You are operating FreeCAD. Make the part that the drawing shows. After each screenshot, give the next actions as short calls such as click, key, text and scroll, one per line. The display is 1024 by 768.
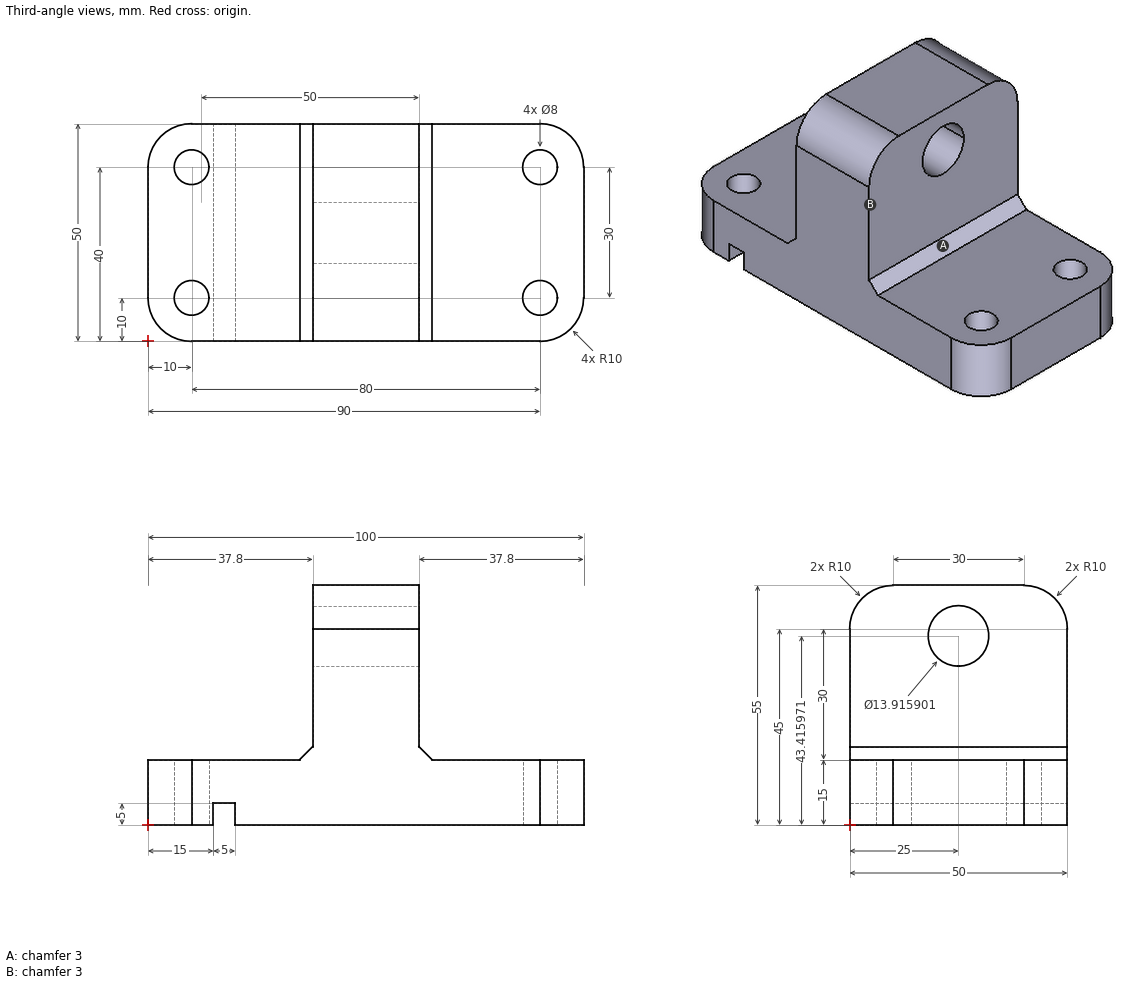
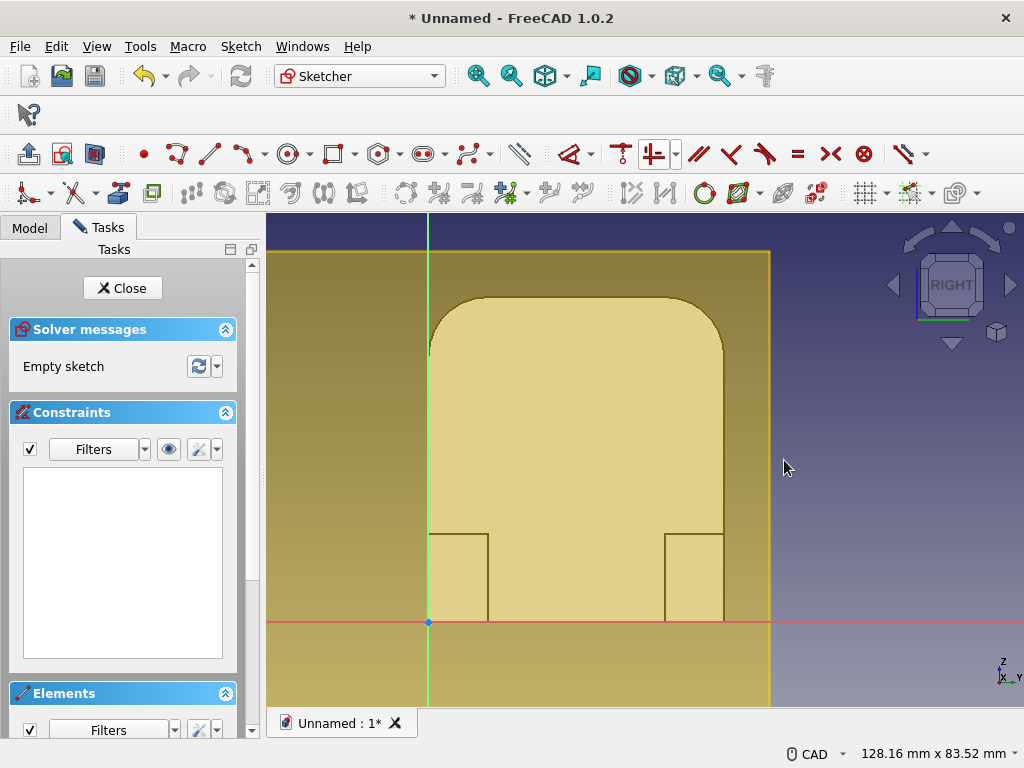
click(177, 154)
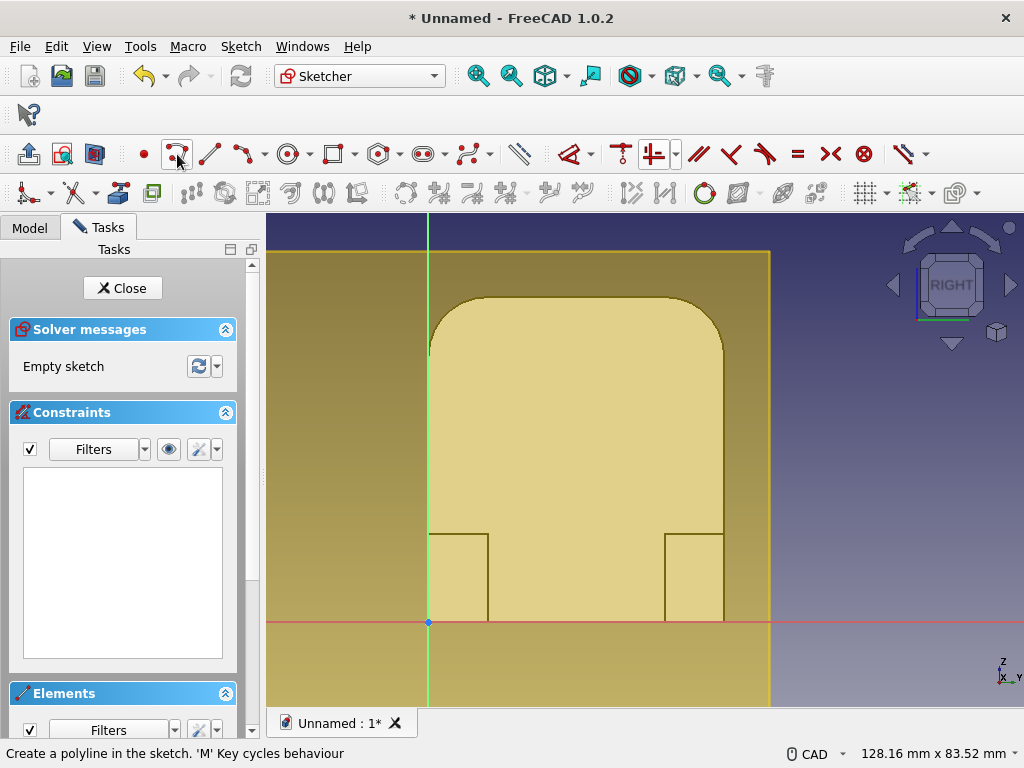
click(724, 356)
click(724, 534)
click(428, 534)
click(437, 356)
right_click(437, 356)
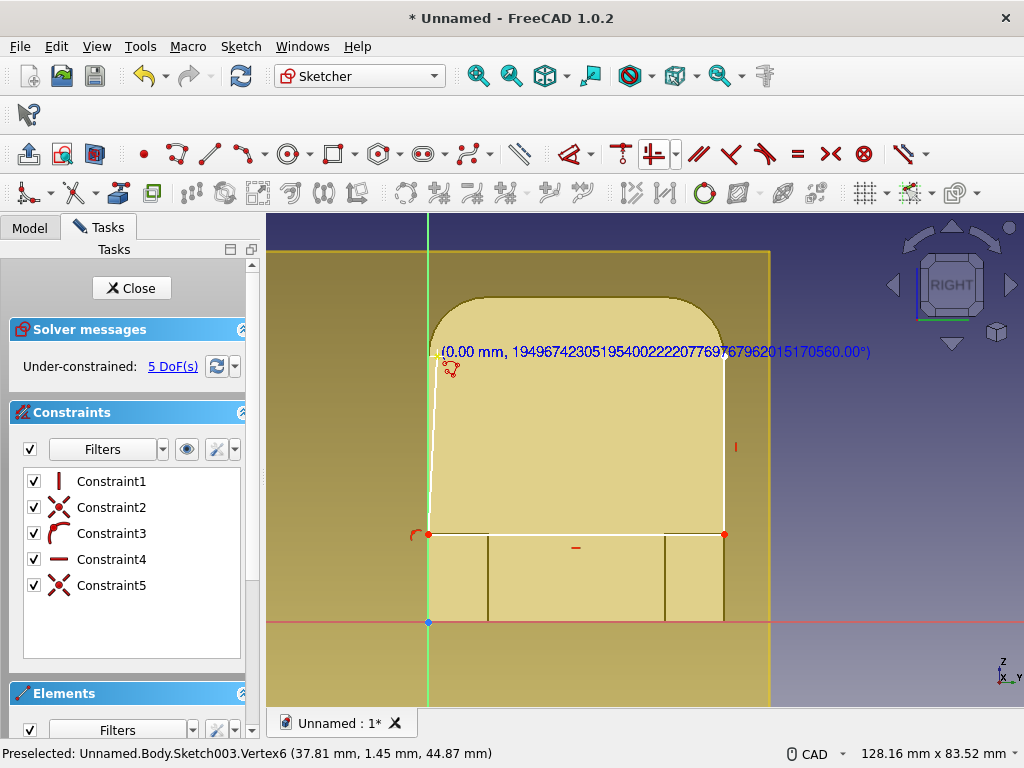
click(210, 154)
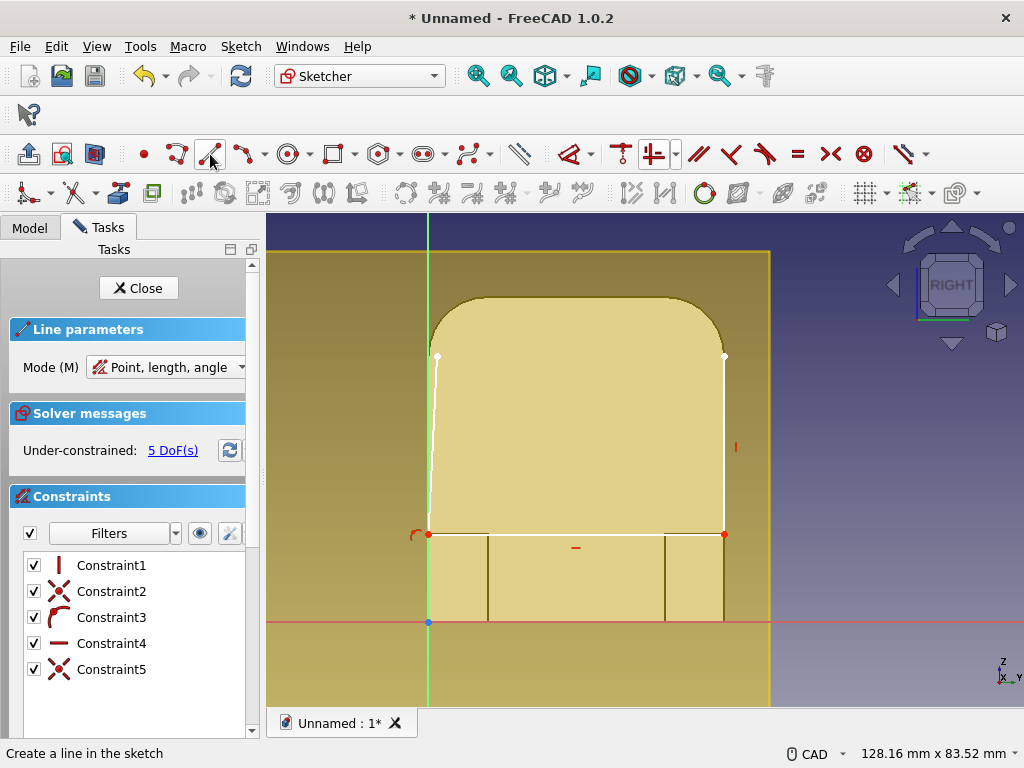
click(488, 297)
click(665, 297)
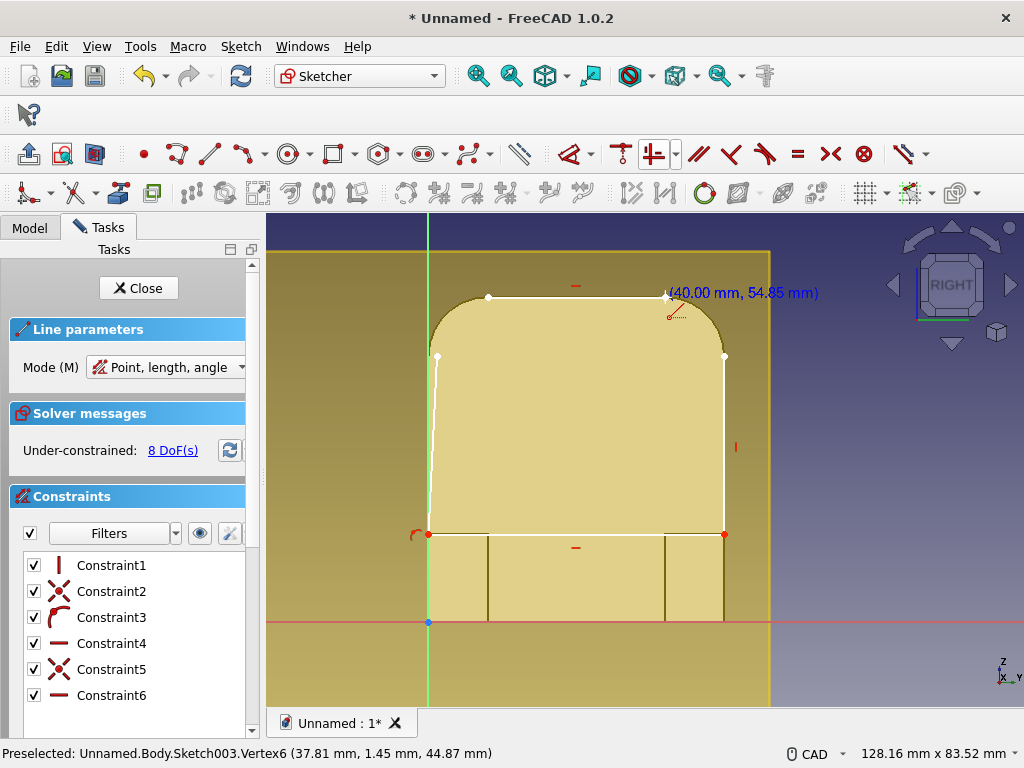
click(242, 154)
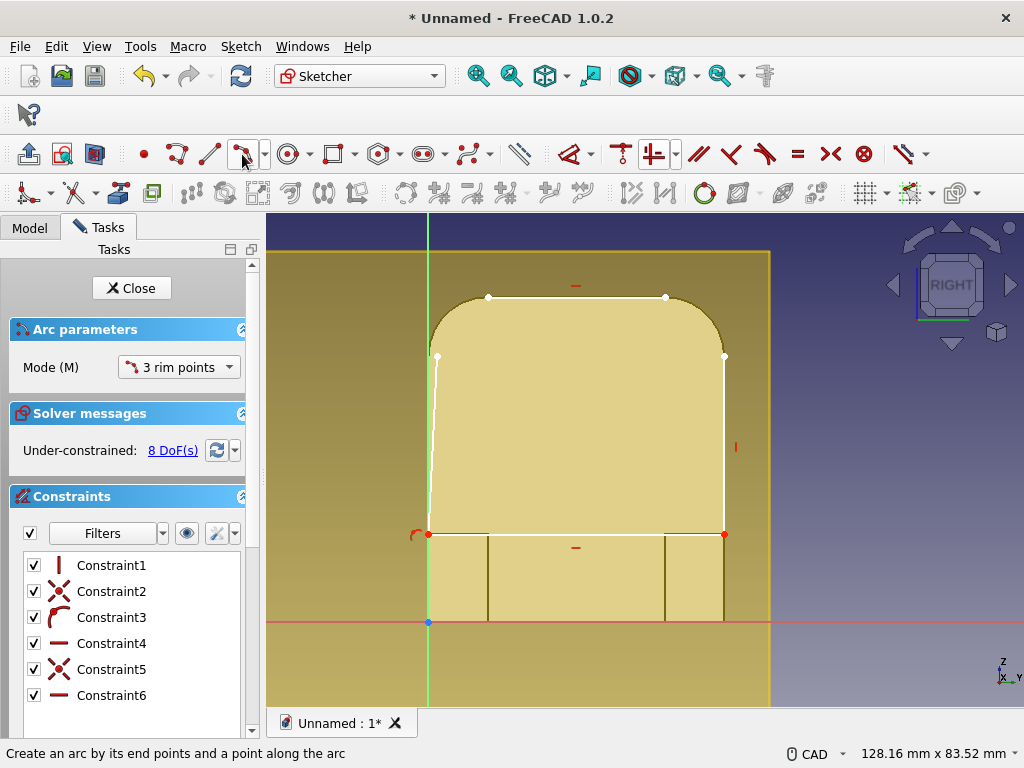
click(437, 357)
click(488, 298)
click(446, 314)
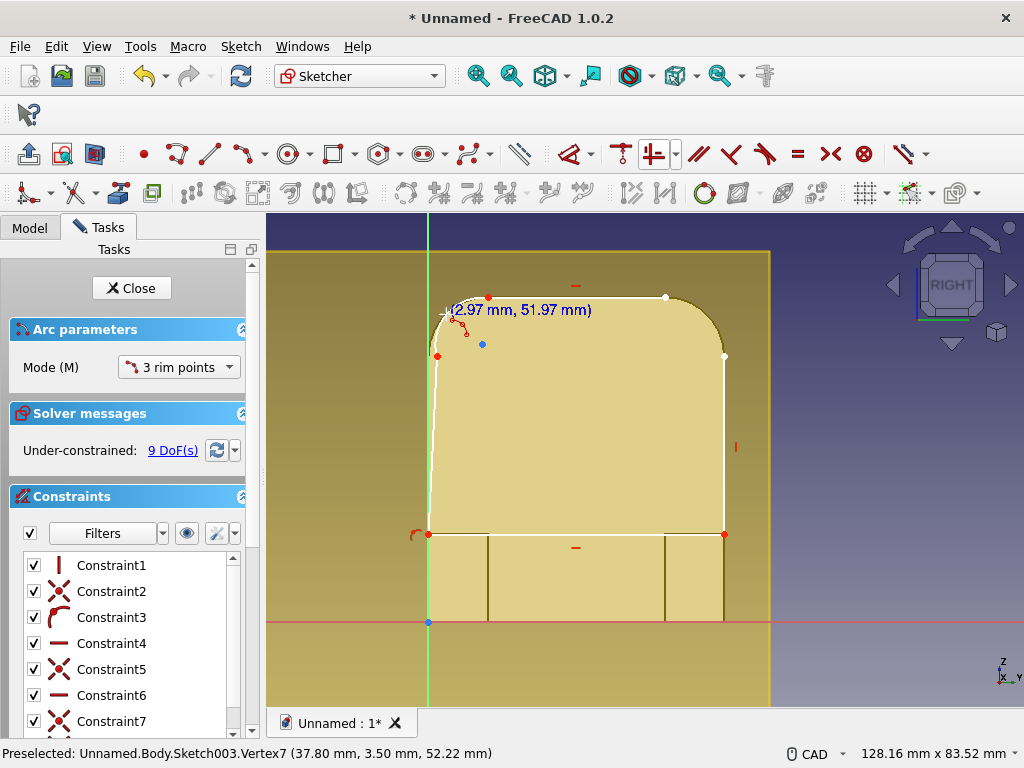
click(665, 298)
click(724, 357)
click(707, 314)
key(Escape)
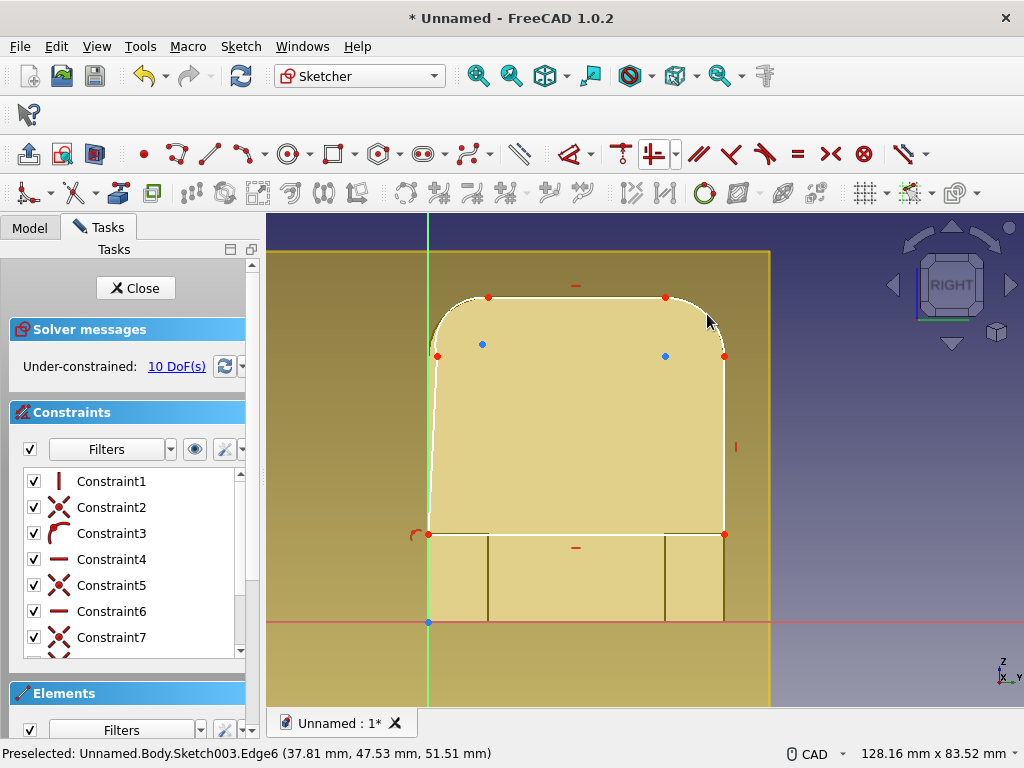
click(724, 410)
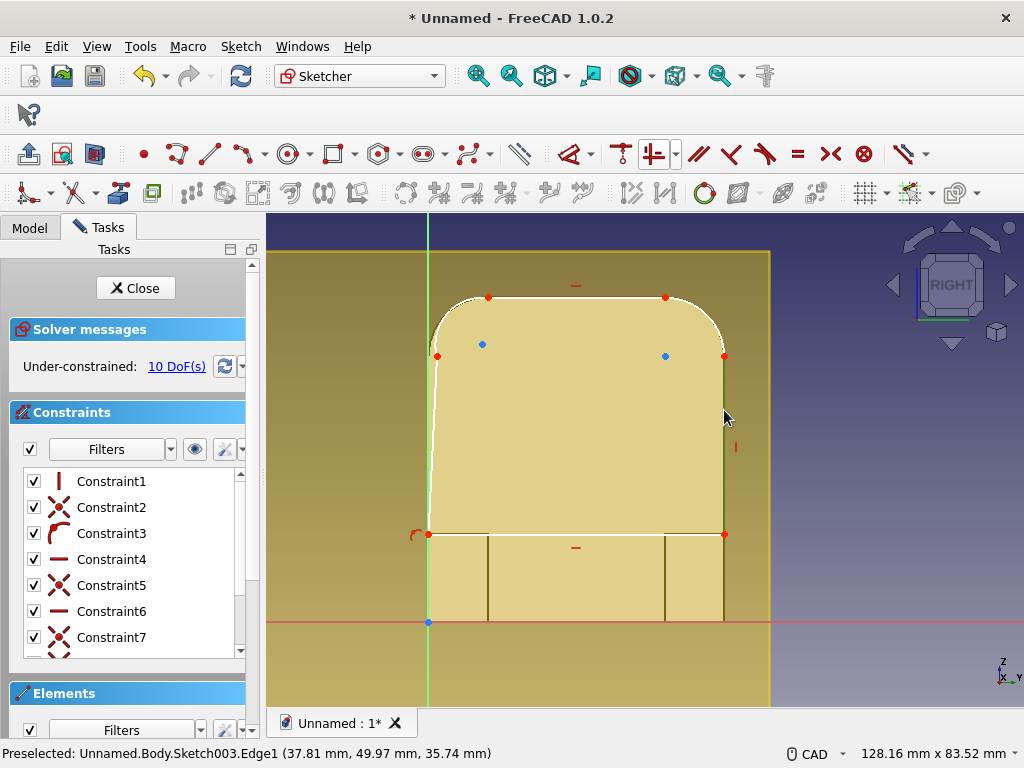
click(718, 330)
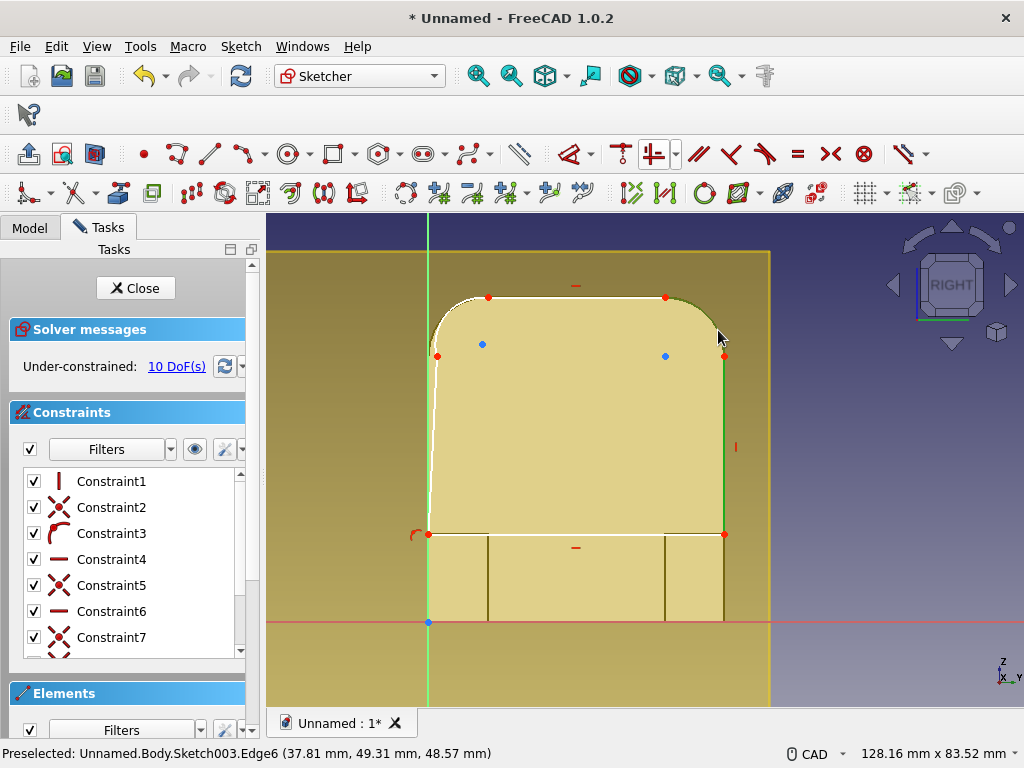
click(765, 154)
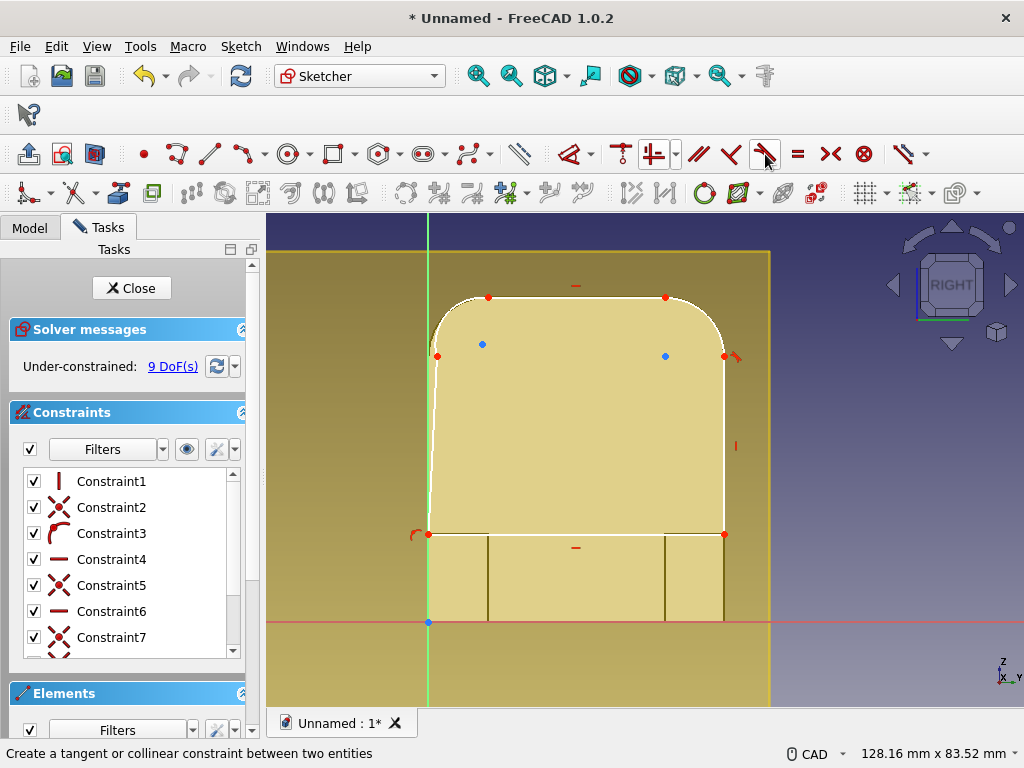
click(431, 482)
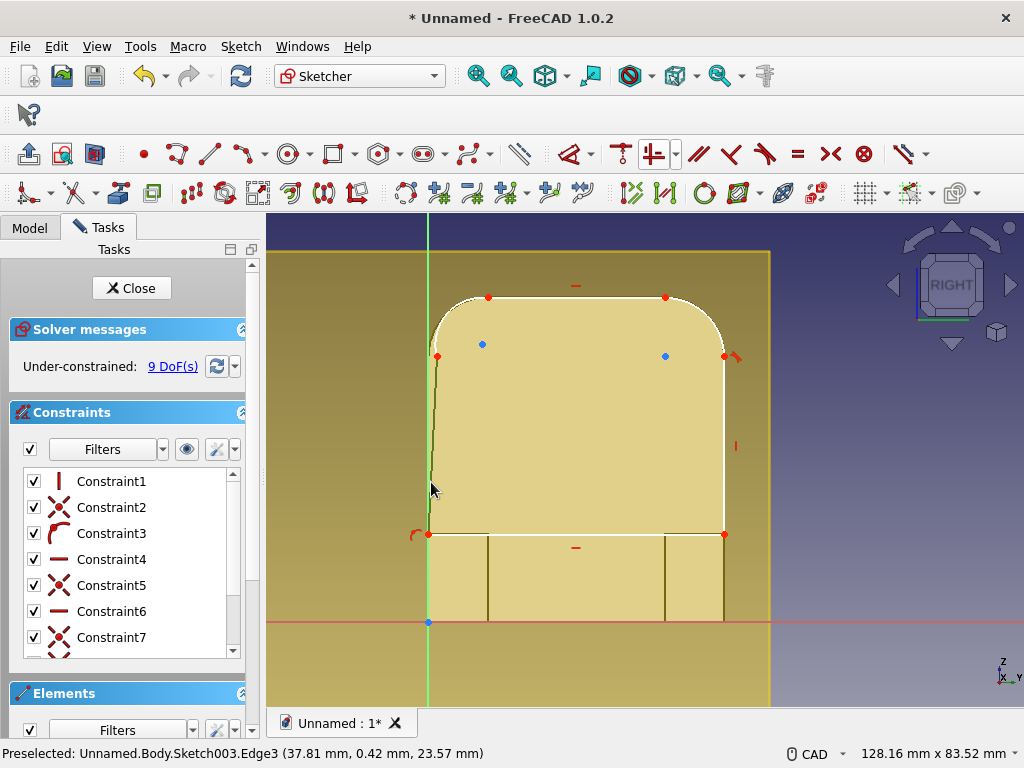
click(461, 303)